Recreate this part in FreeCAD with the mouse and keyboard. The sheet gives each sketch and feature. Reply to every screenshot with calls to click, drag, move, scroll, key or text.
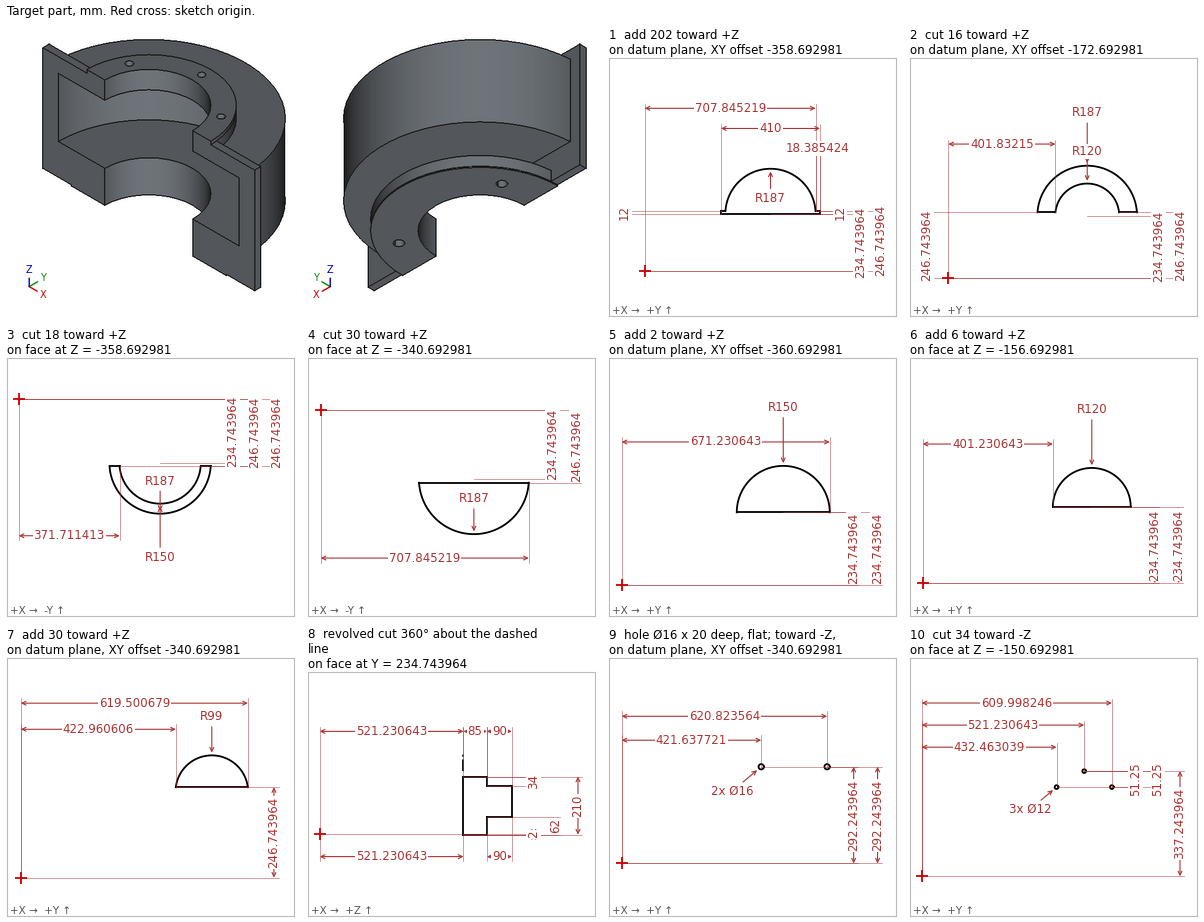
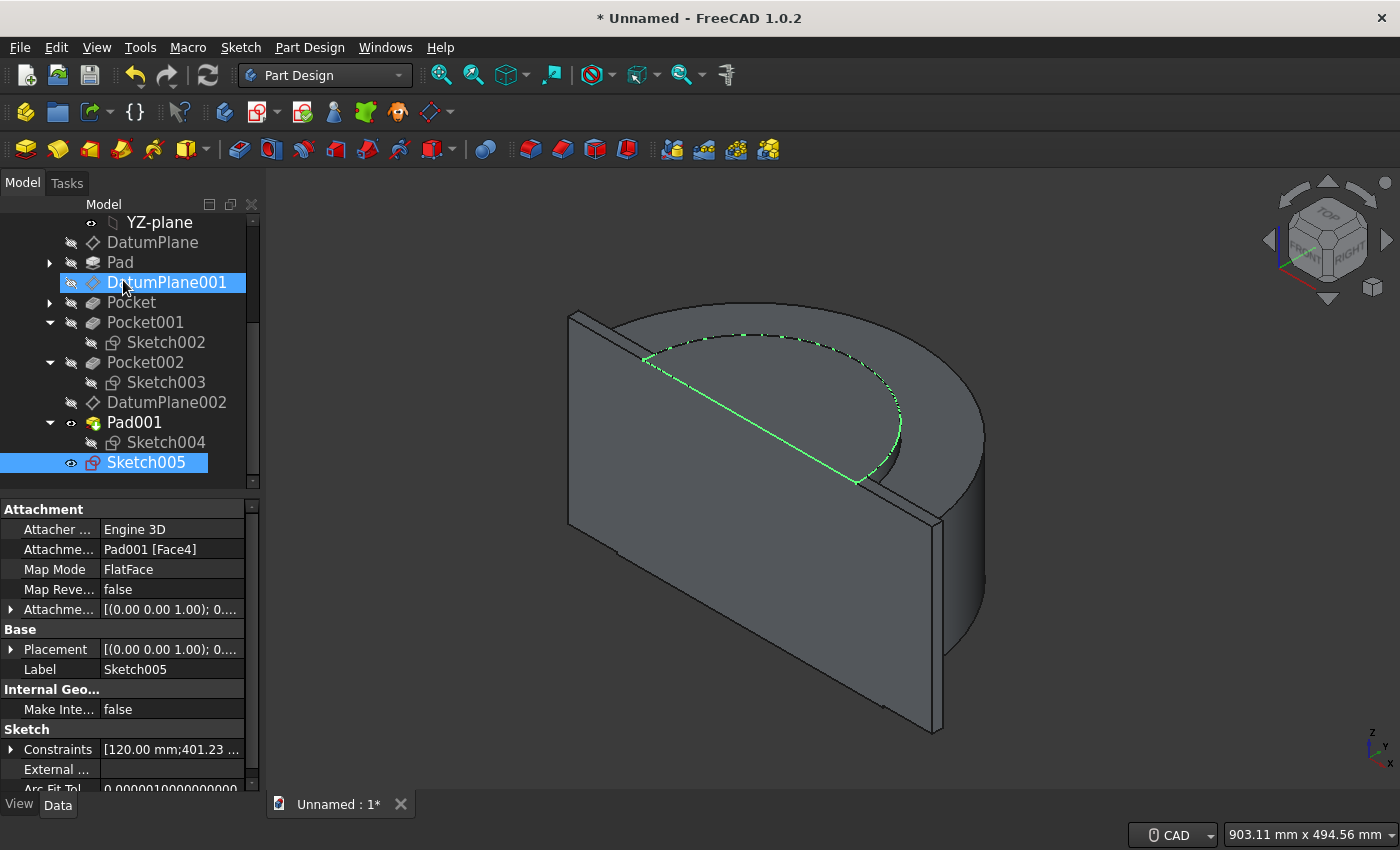
click(26, 150)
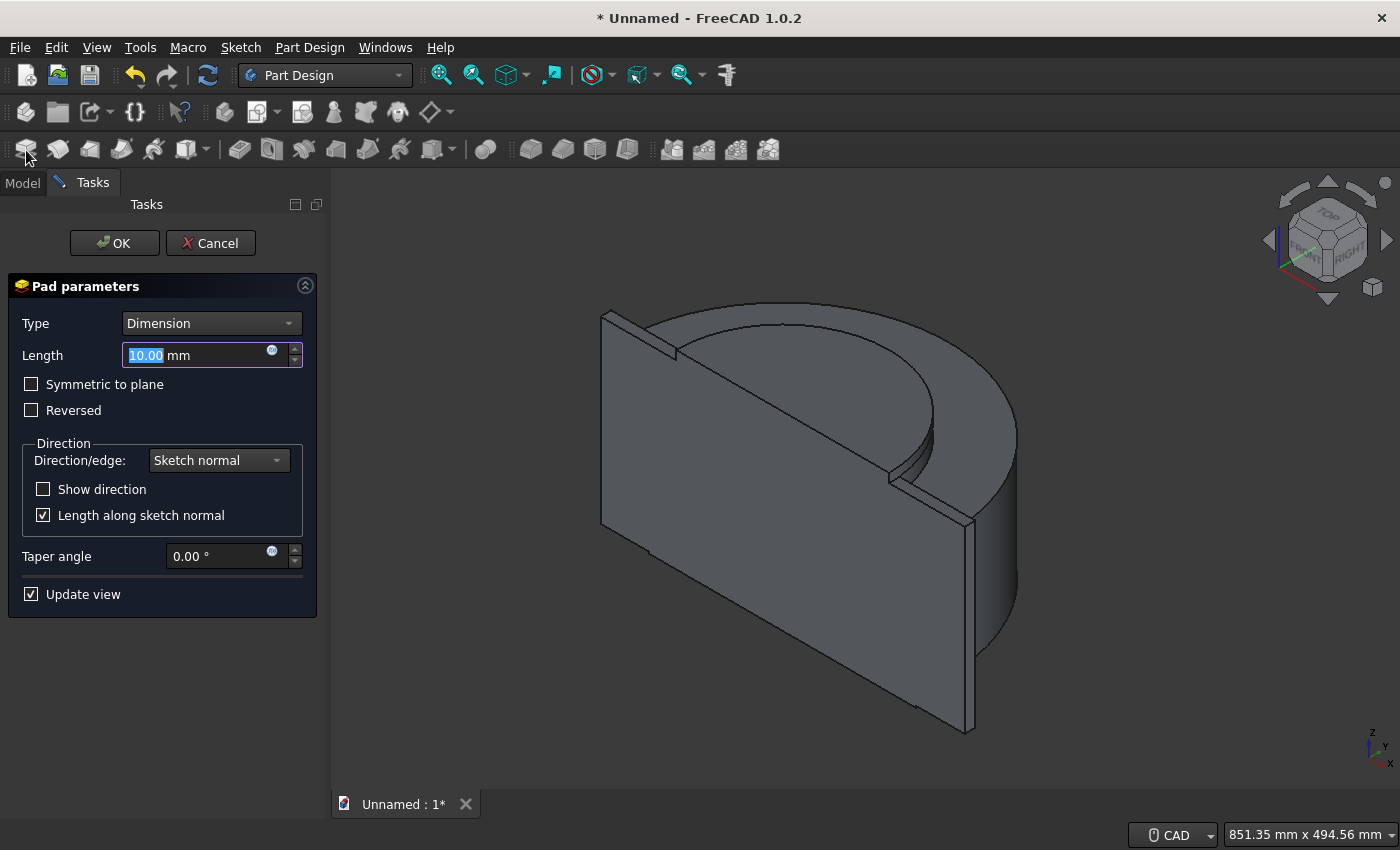
text(6)
key(Tab)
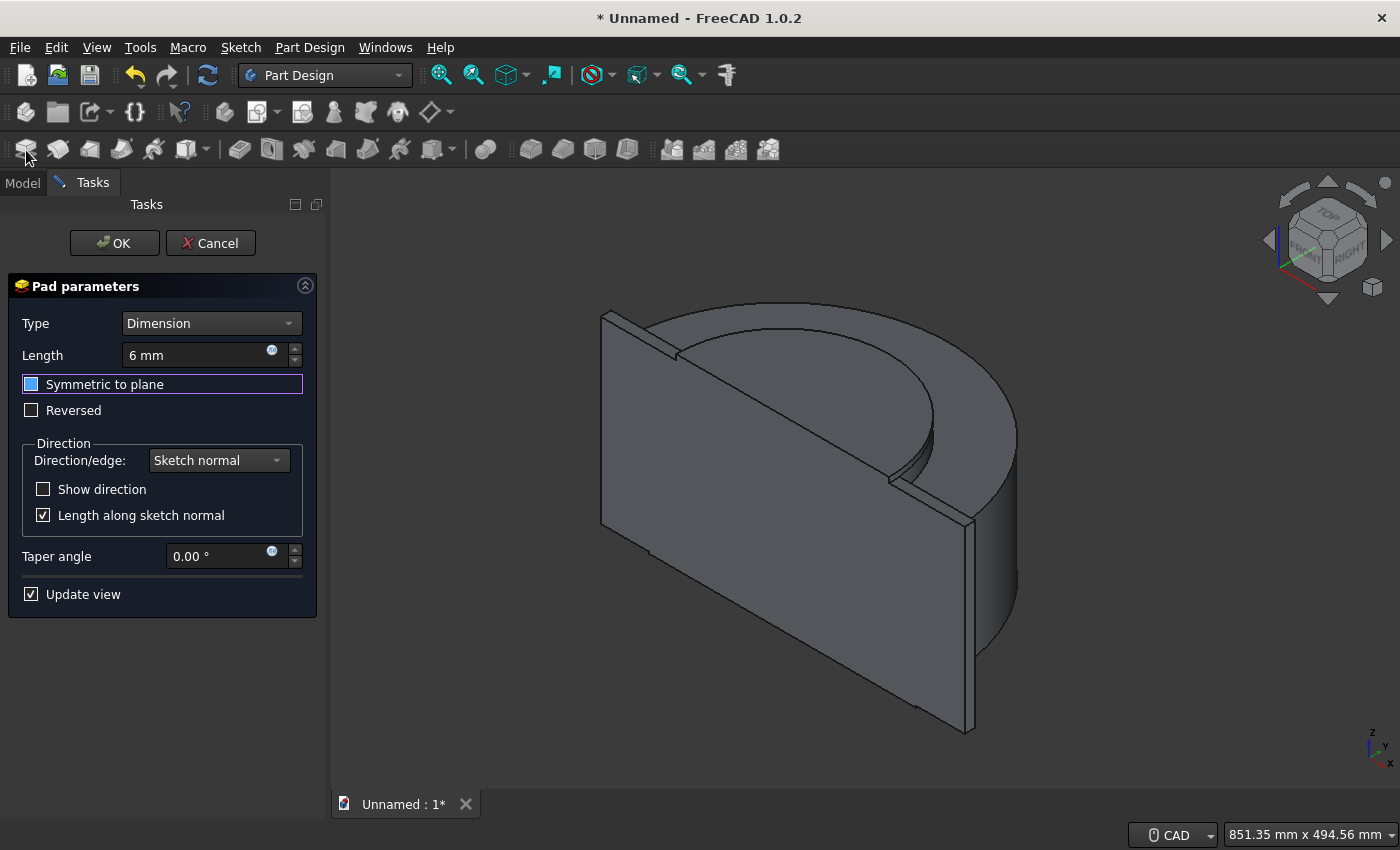
click(115, 243)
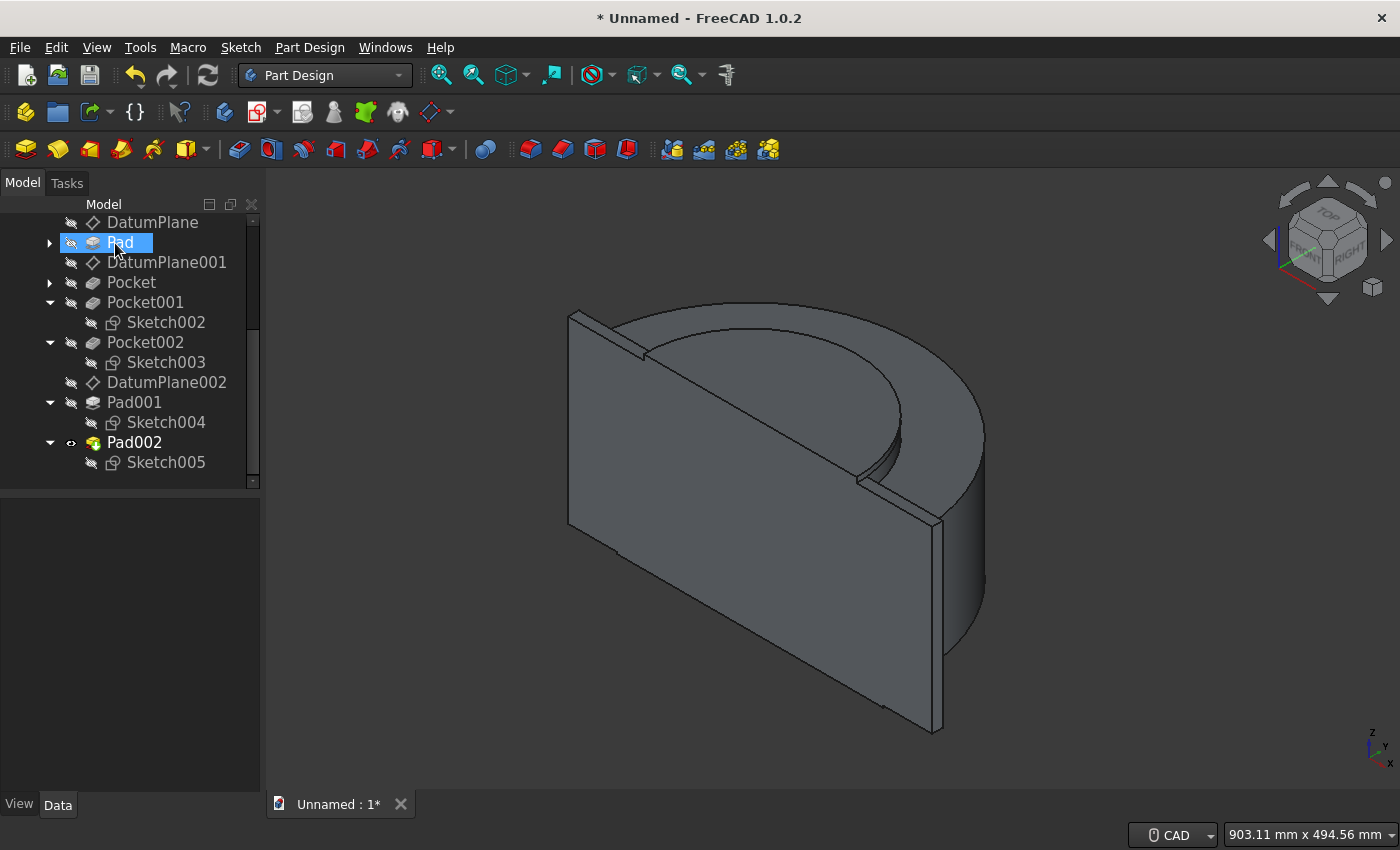
scroll(140, 338, down, 3)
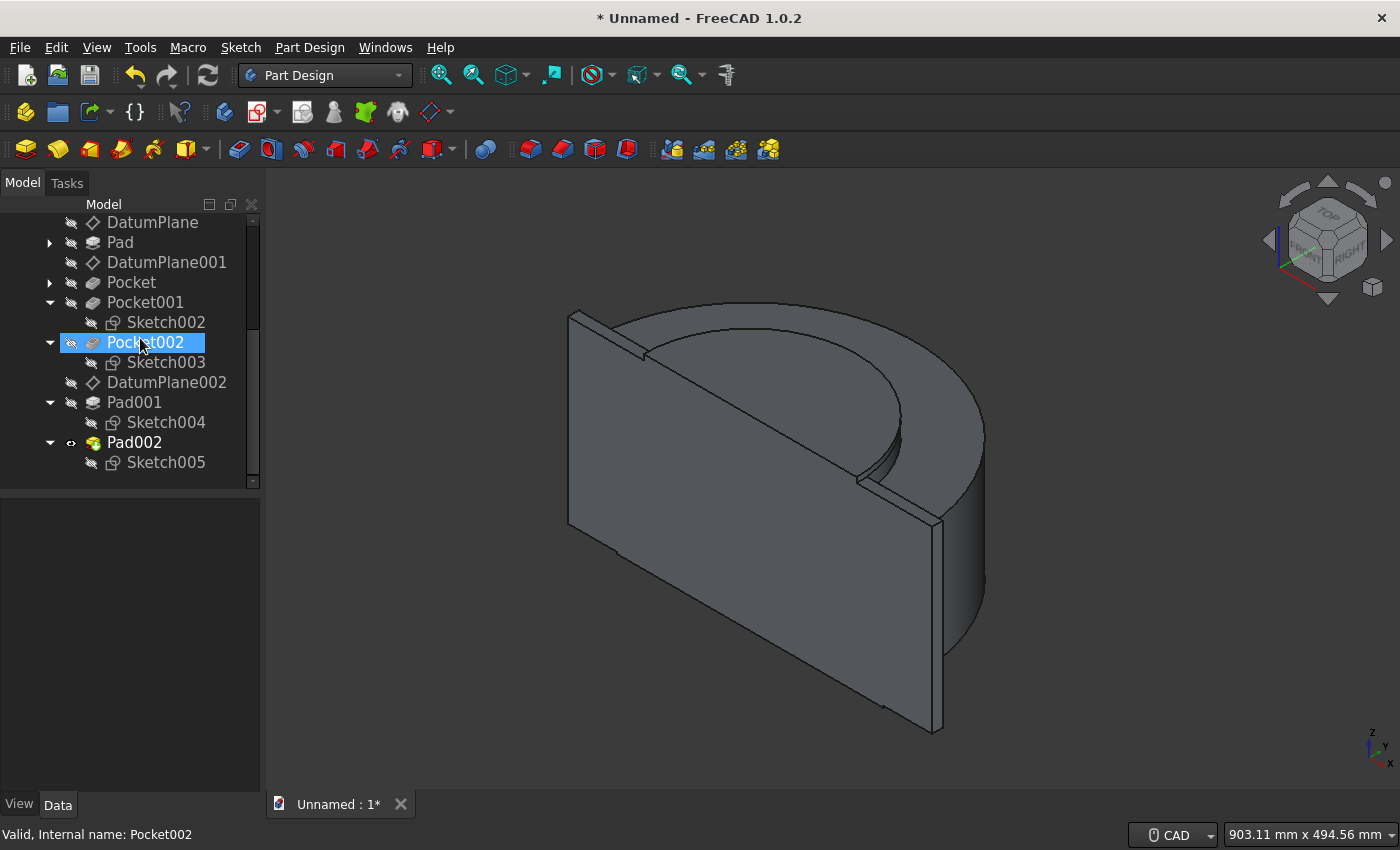
scroll(140, 338, up, 15)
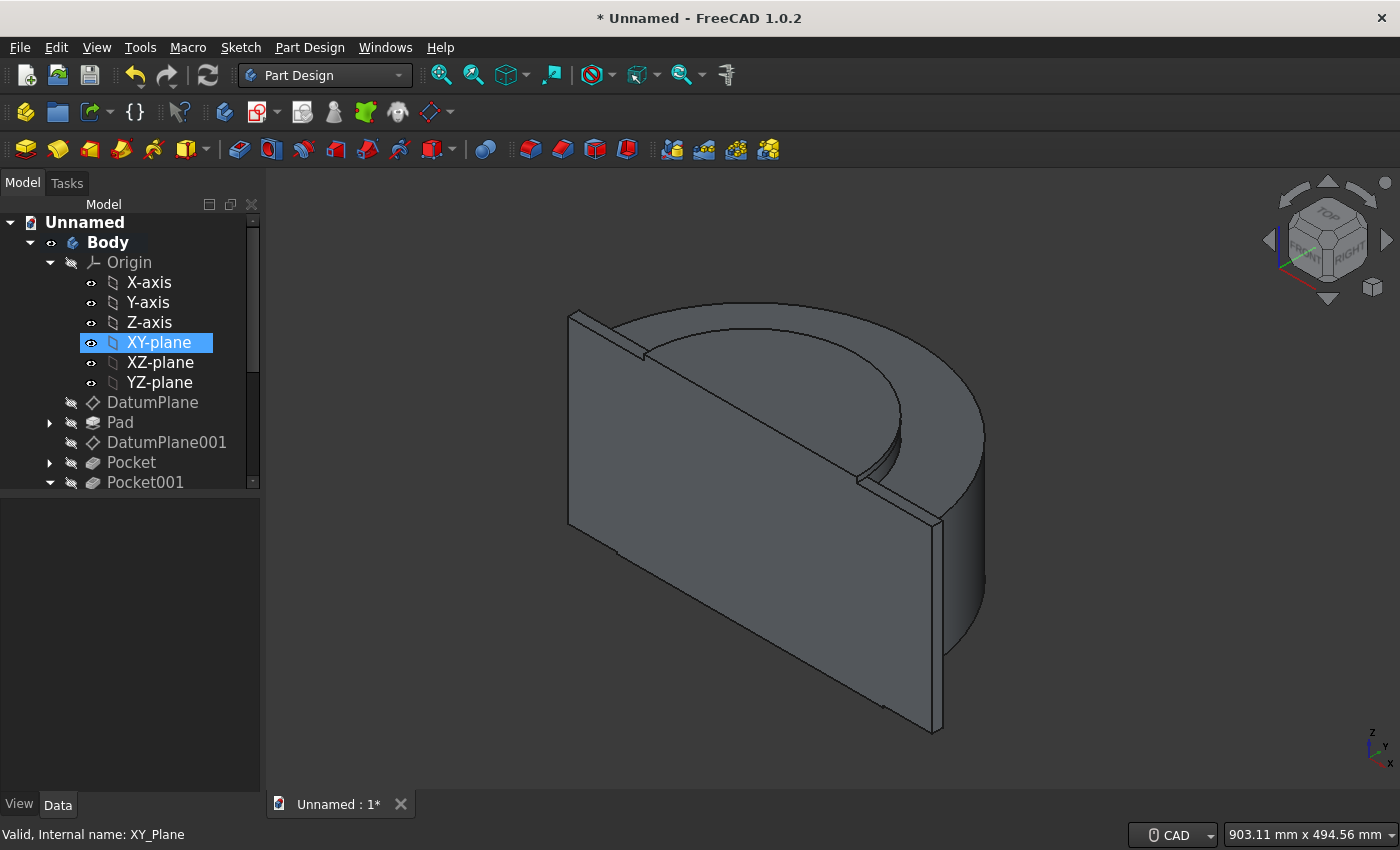
click(136, 343)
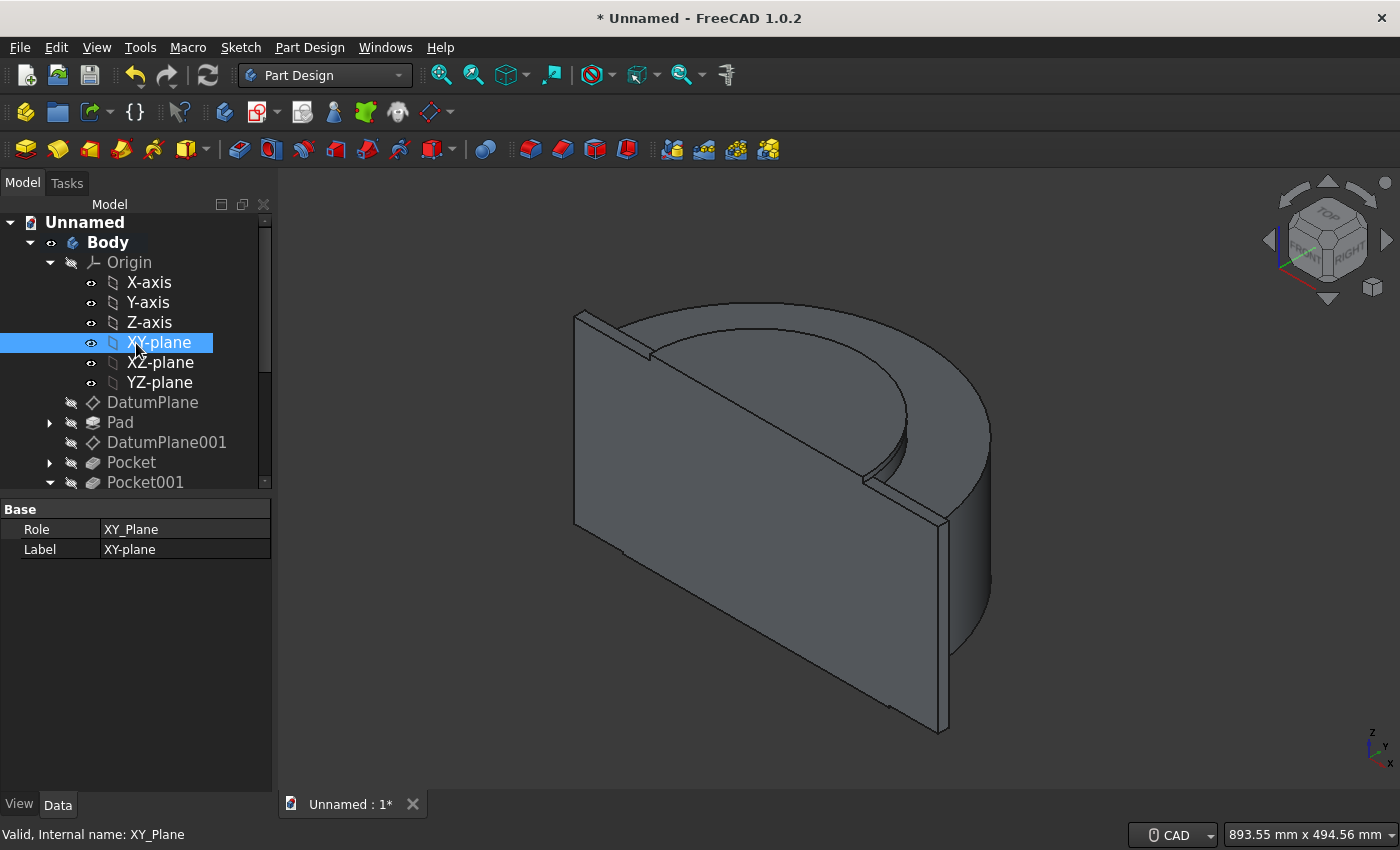
click(430, 112)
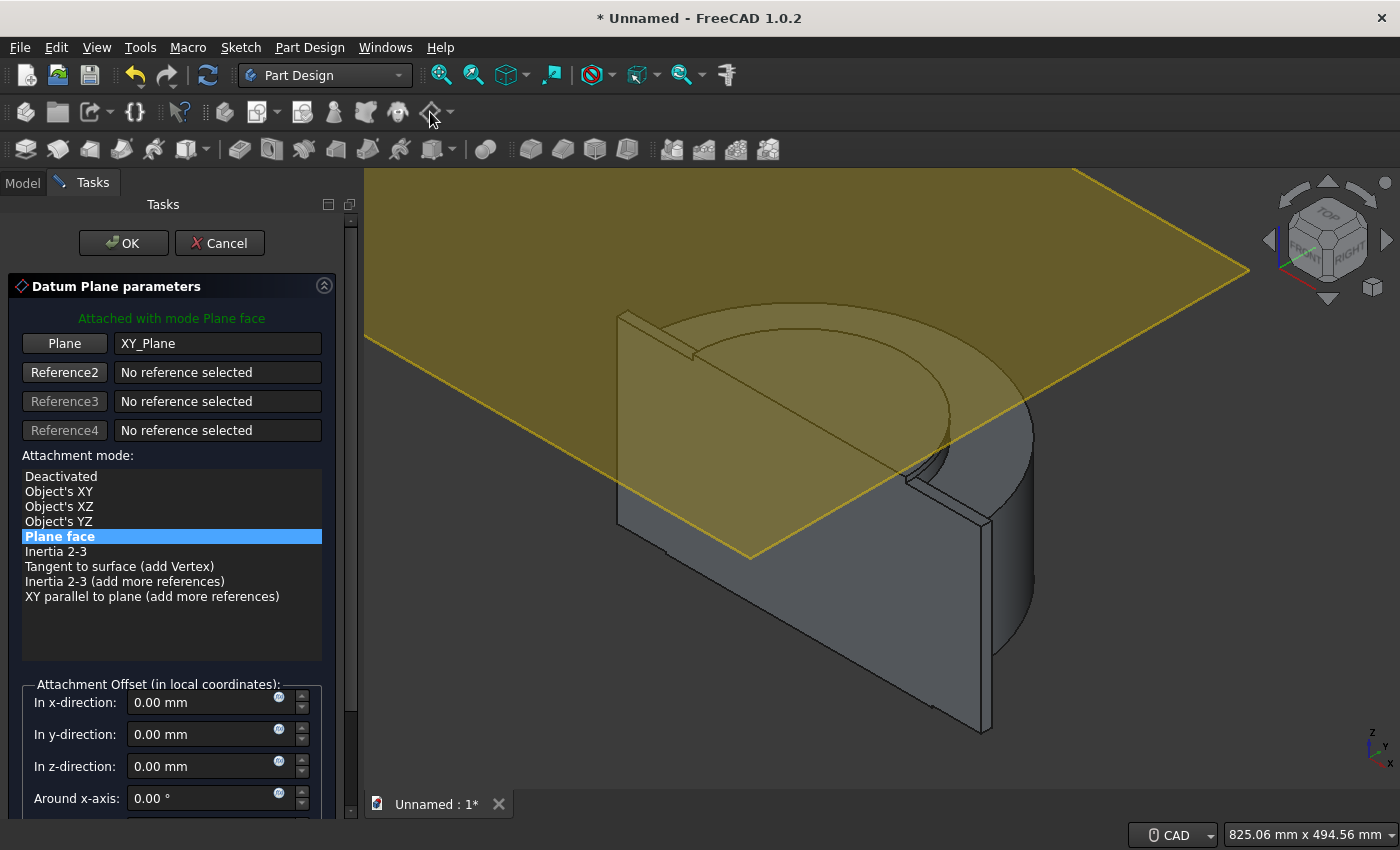
triple_click(210, 766)